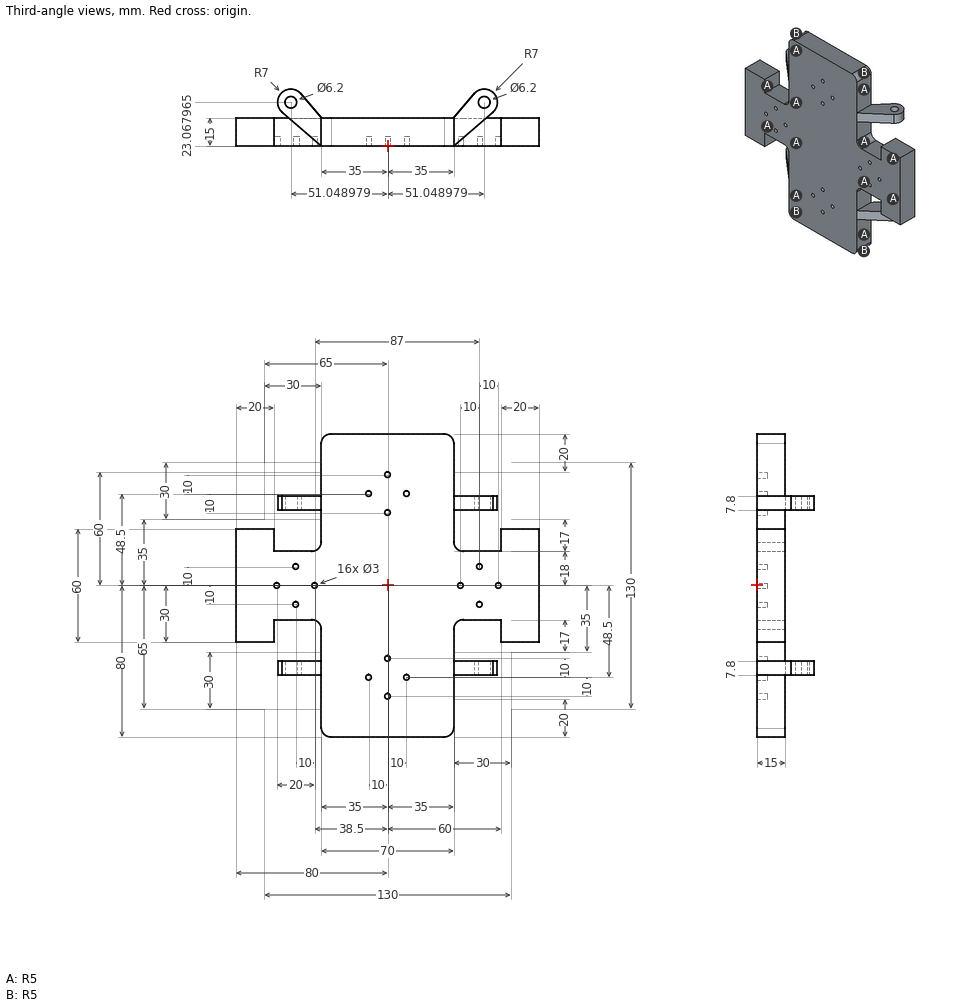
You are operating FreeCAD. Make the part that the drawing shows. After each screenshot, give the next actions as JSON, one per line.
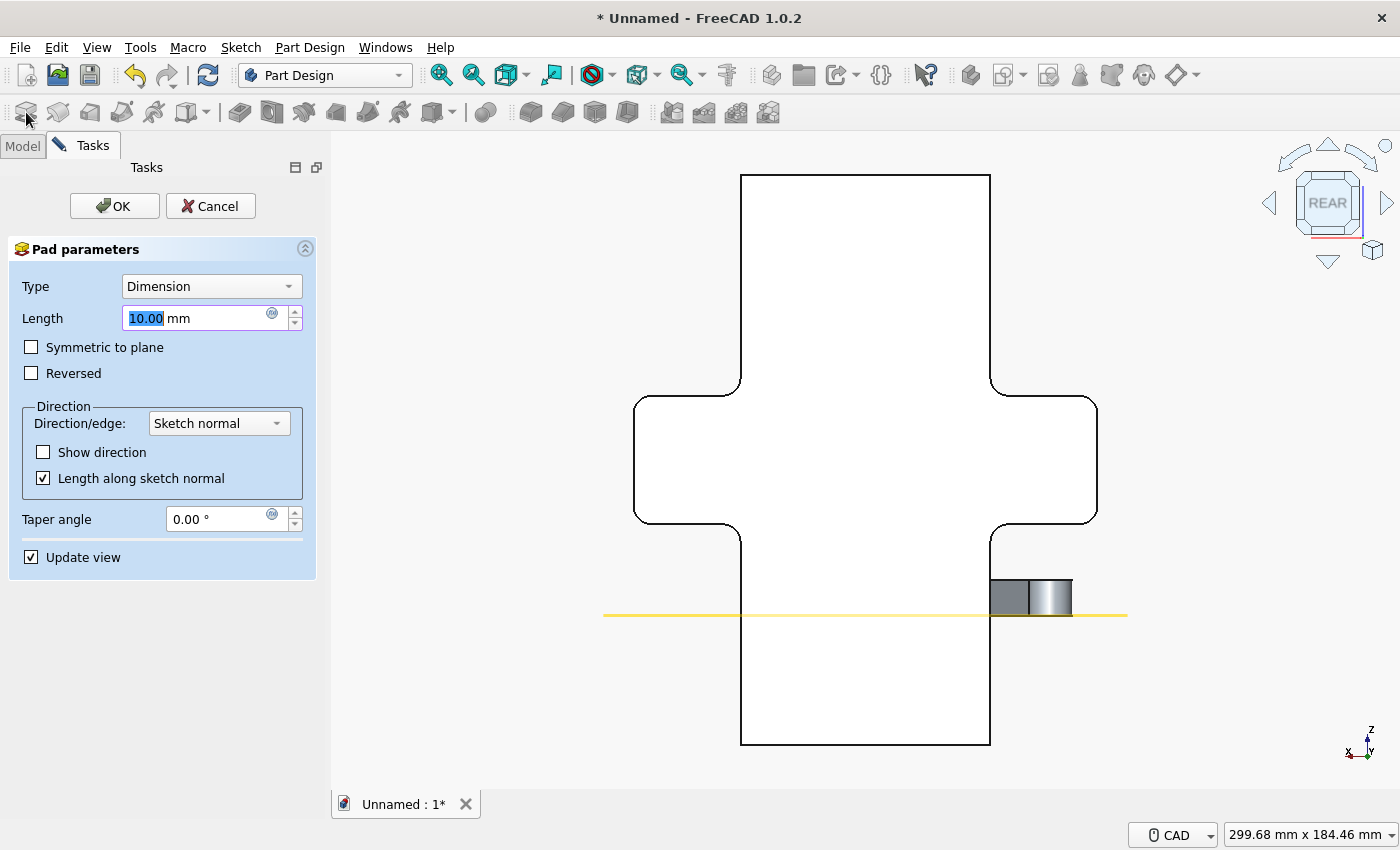
{"action": "type", "text": "7.8"}
{"action": "key", "text": "Tab"}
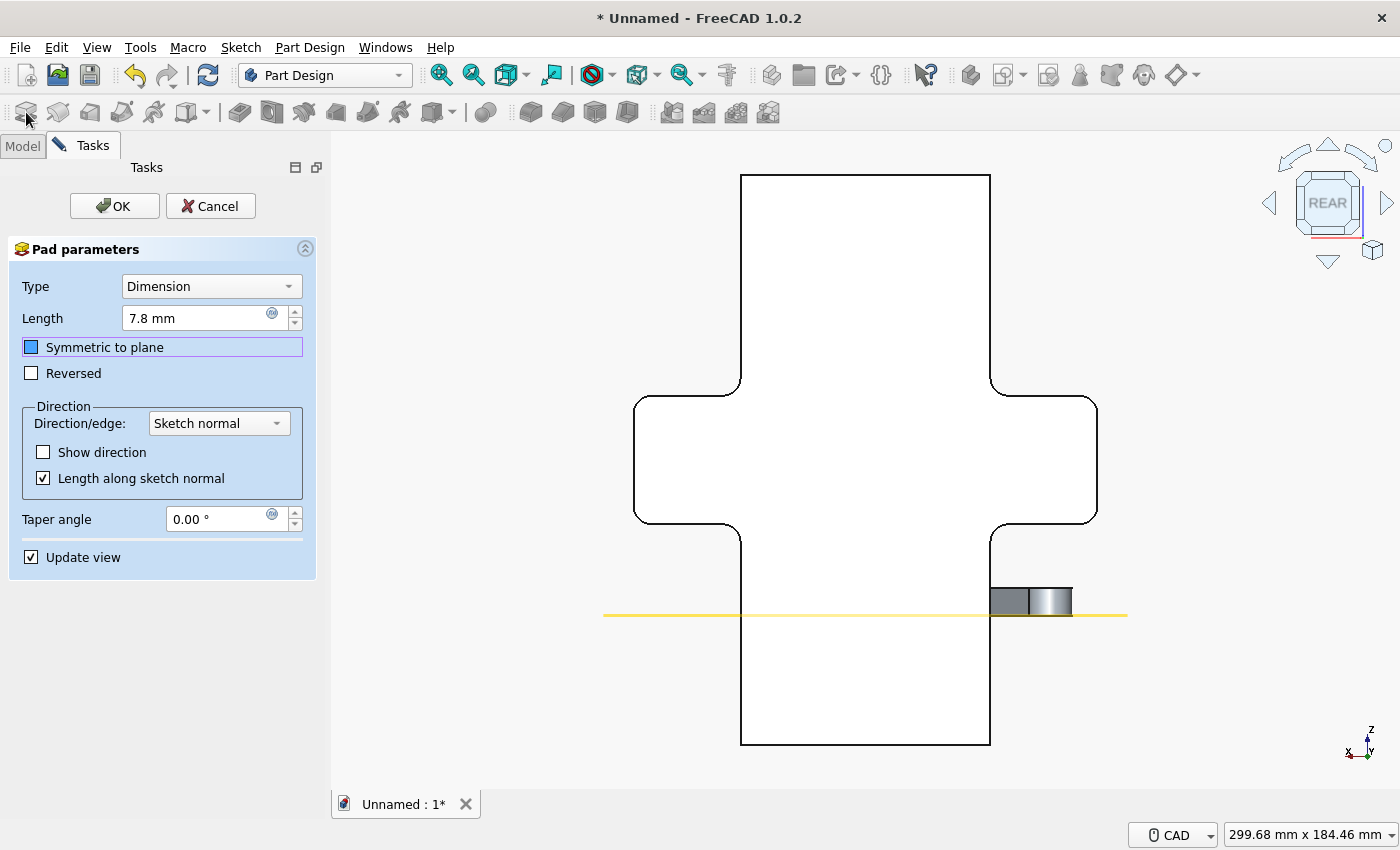
{"action": "left_click", "coordinate": [30, 347]}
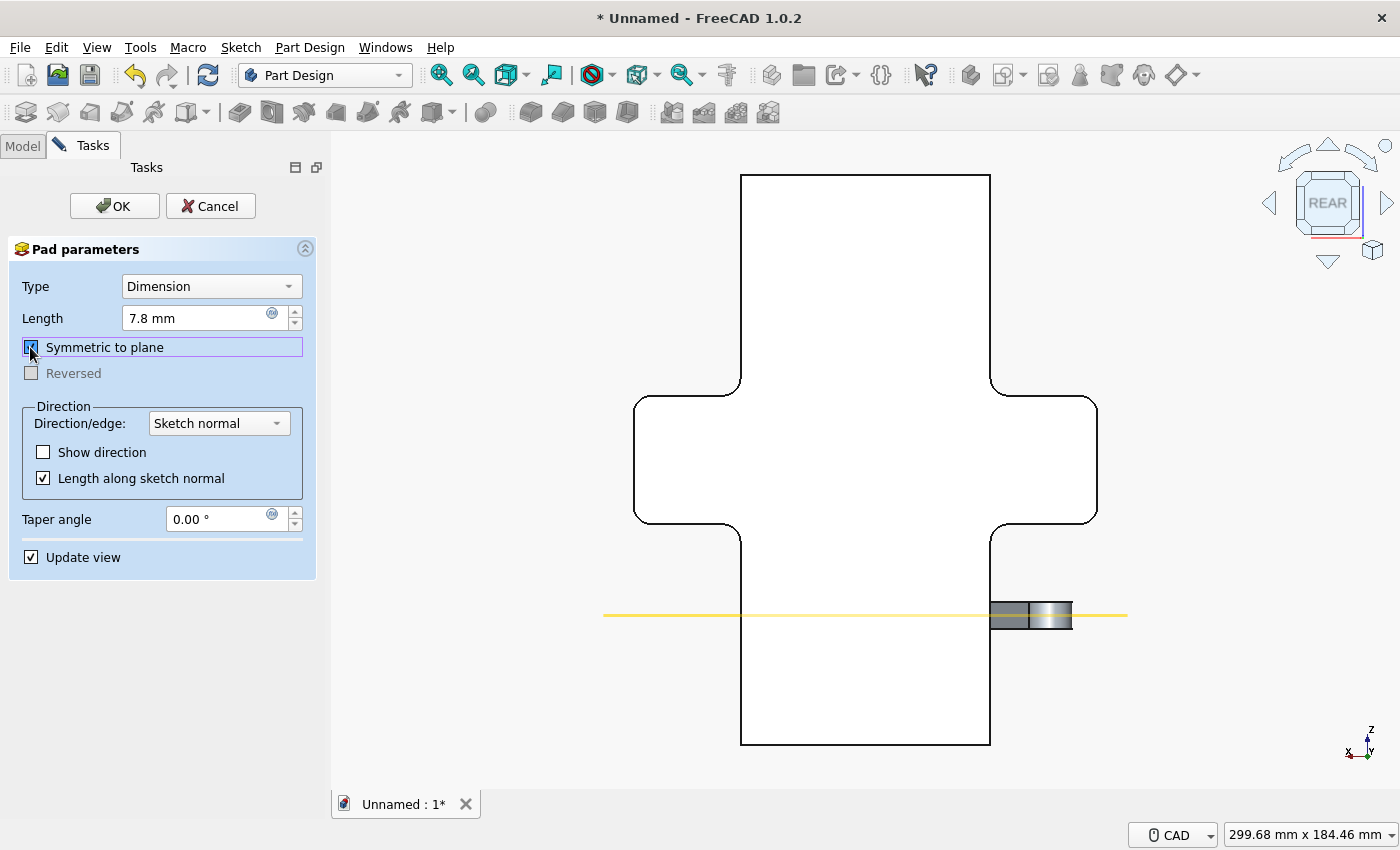
{"action": "left_click", "coordinate": [115, 206]}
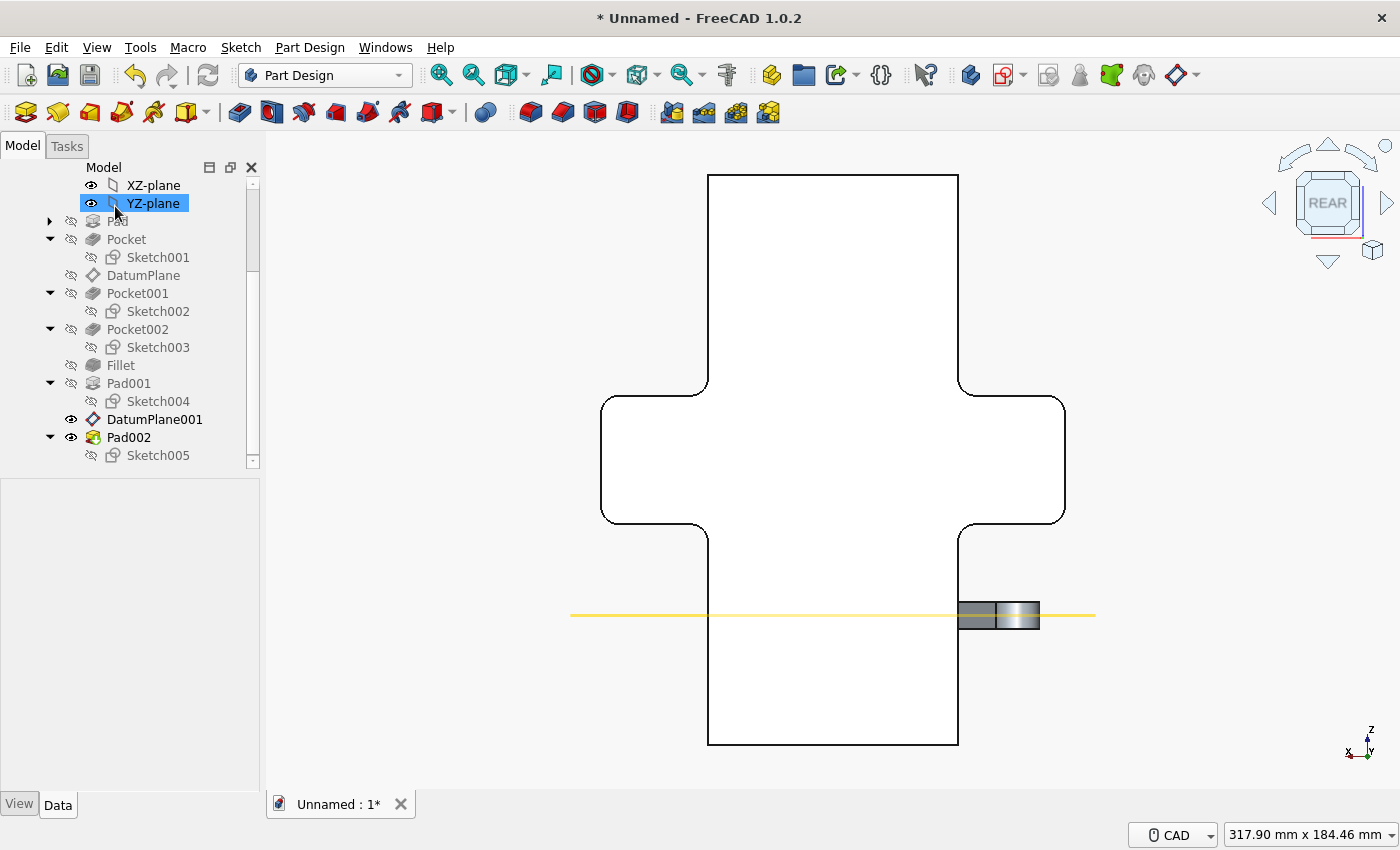
{"action": "left_click", "coordinate": [116, 419]}
{"action": "key", "text": "space"}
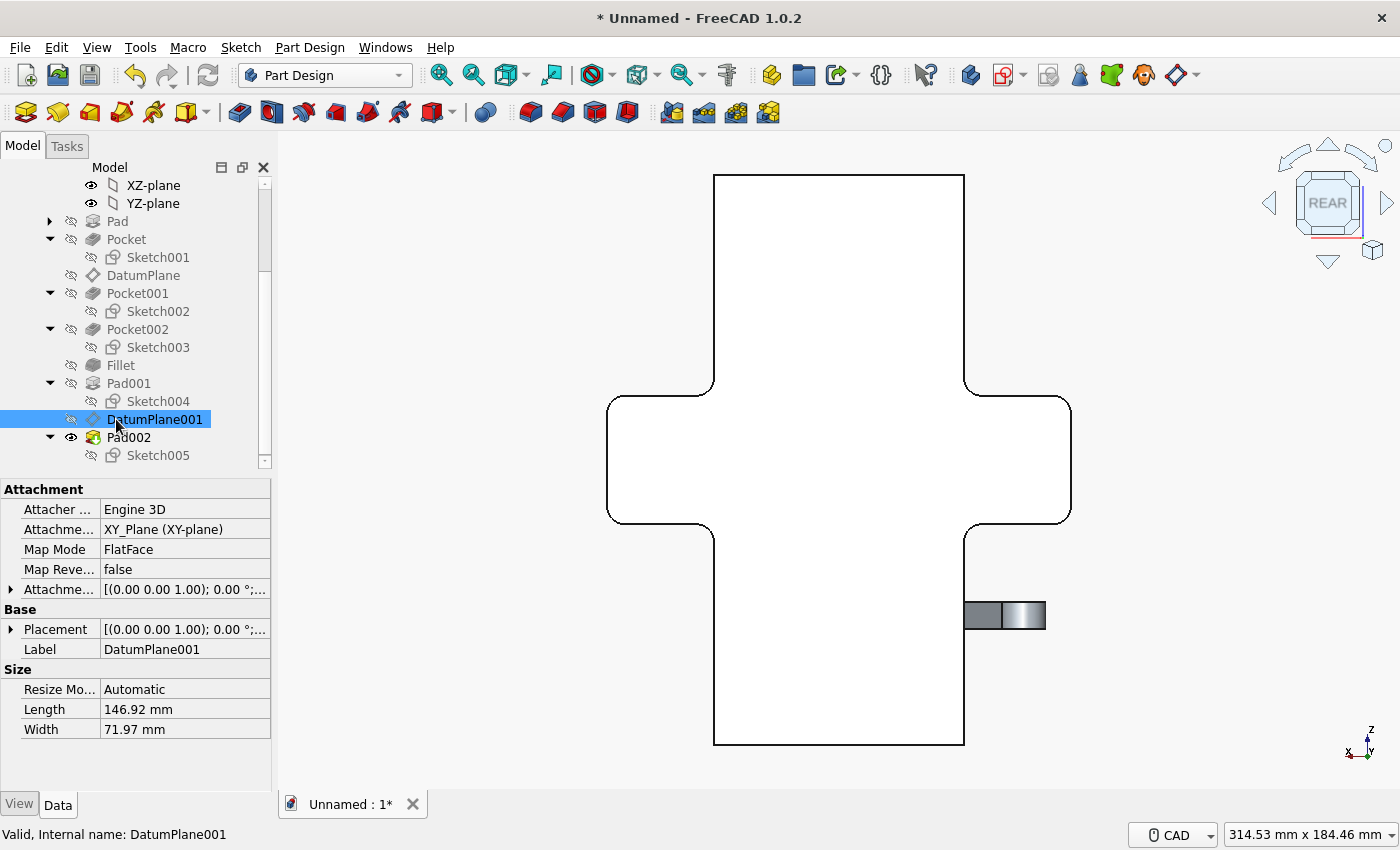
{"action": "left_click", "coordinate": [116, 437]}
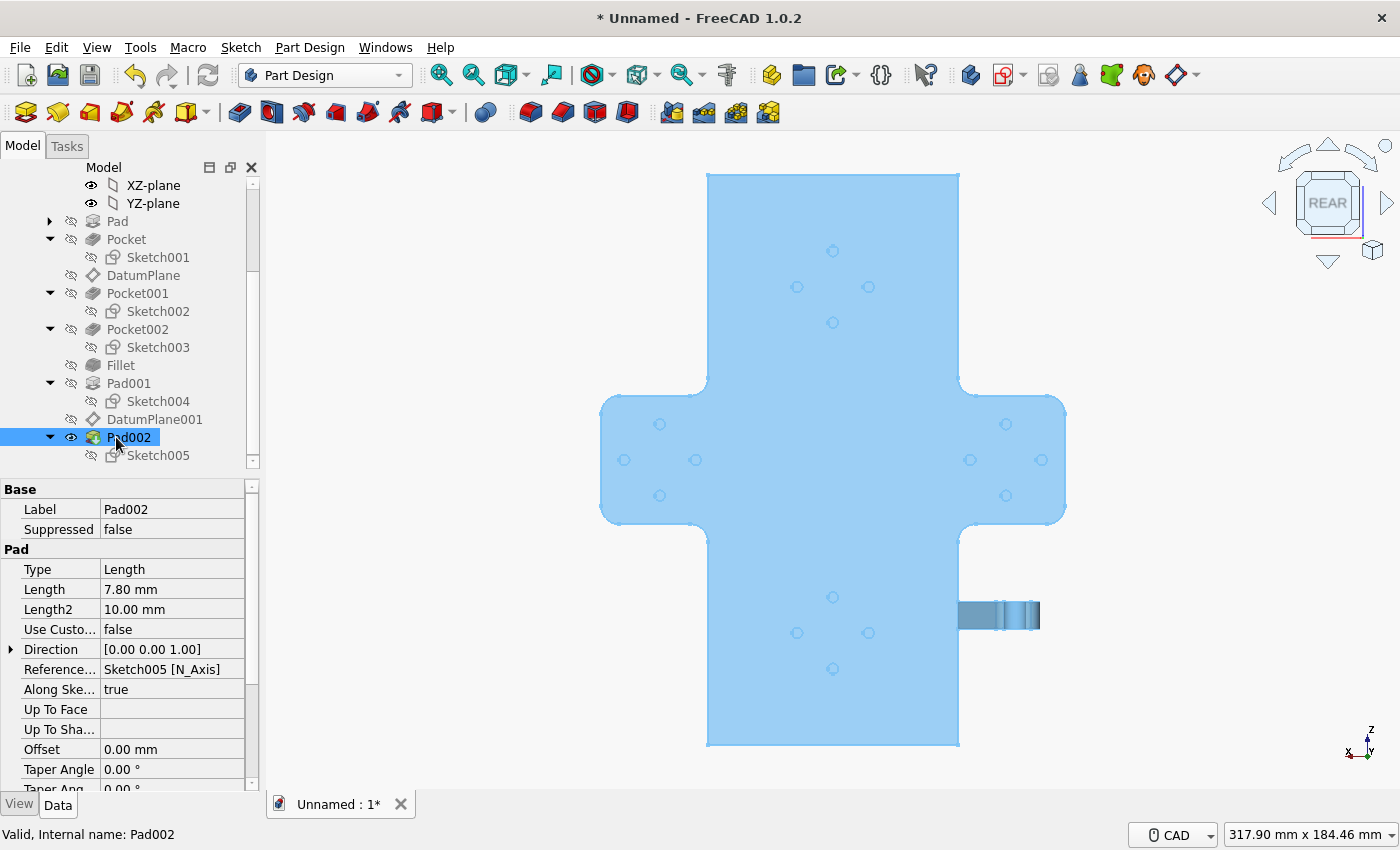
{"action": "left_click", "coordinate": [672, 112]}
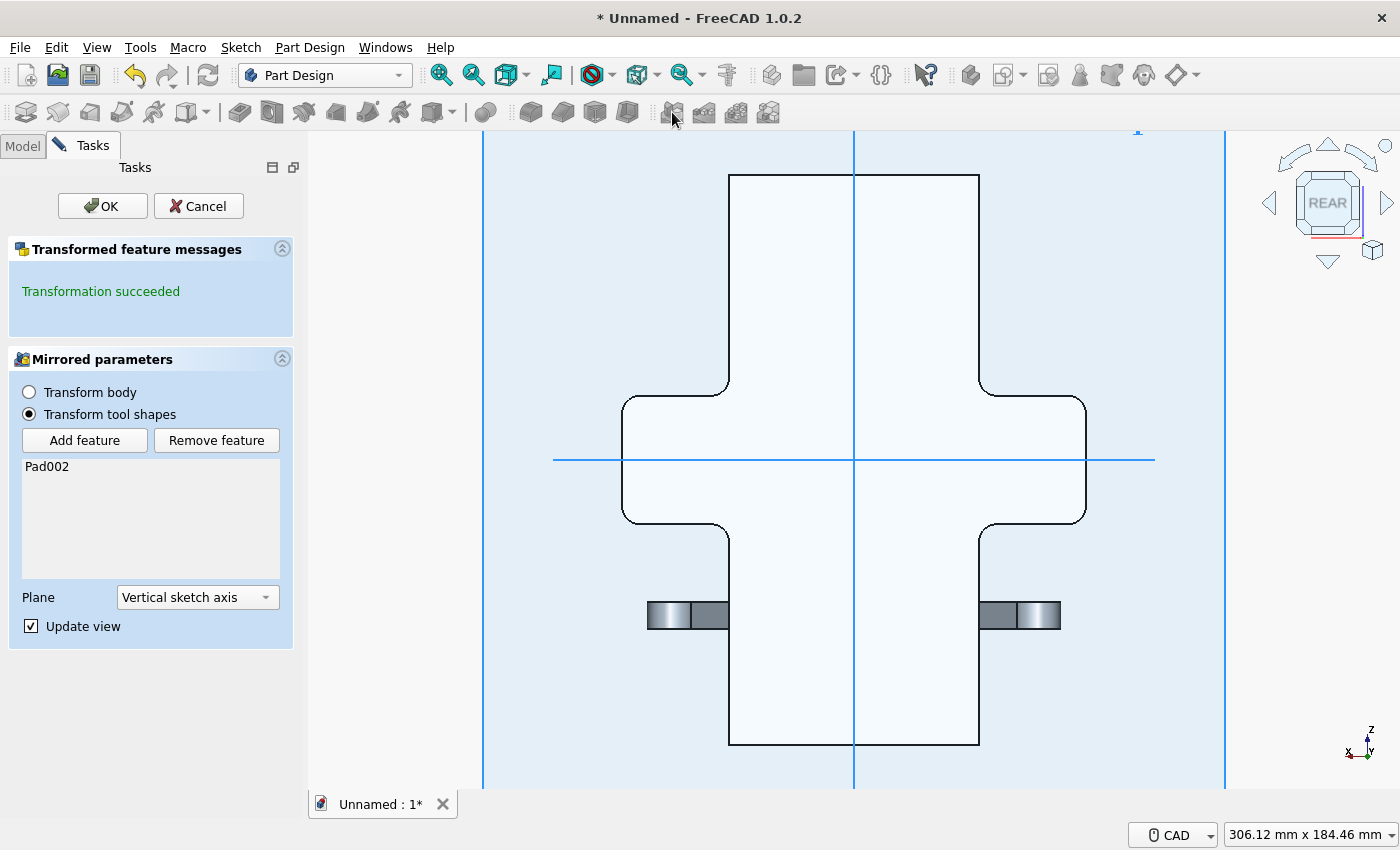
{"action": "left_click", "coordinate": [198, 598]}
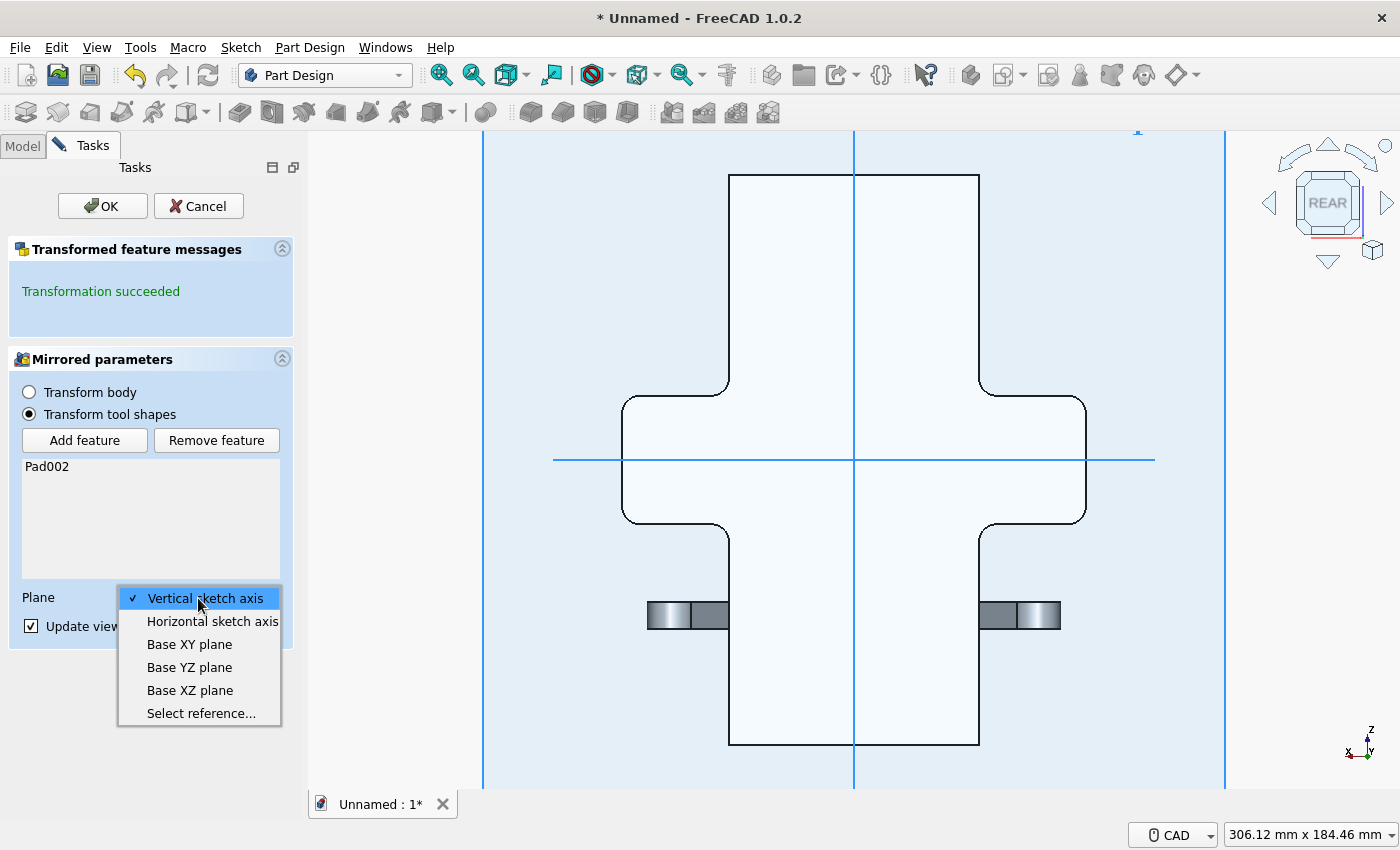
{"action": "left_click", "coordinate": [198, 668]}